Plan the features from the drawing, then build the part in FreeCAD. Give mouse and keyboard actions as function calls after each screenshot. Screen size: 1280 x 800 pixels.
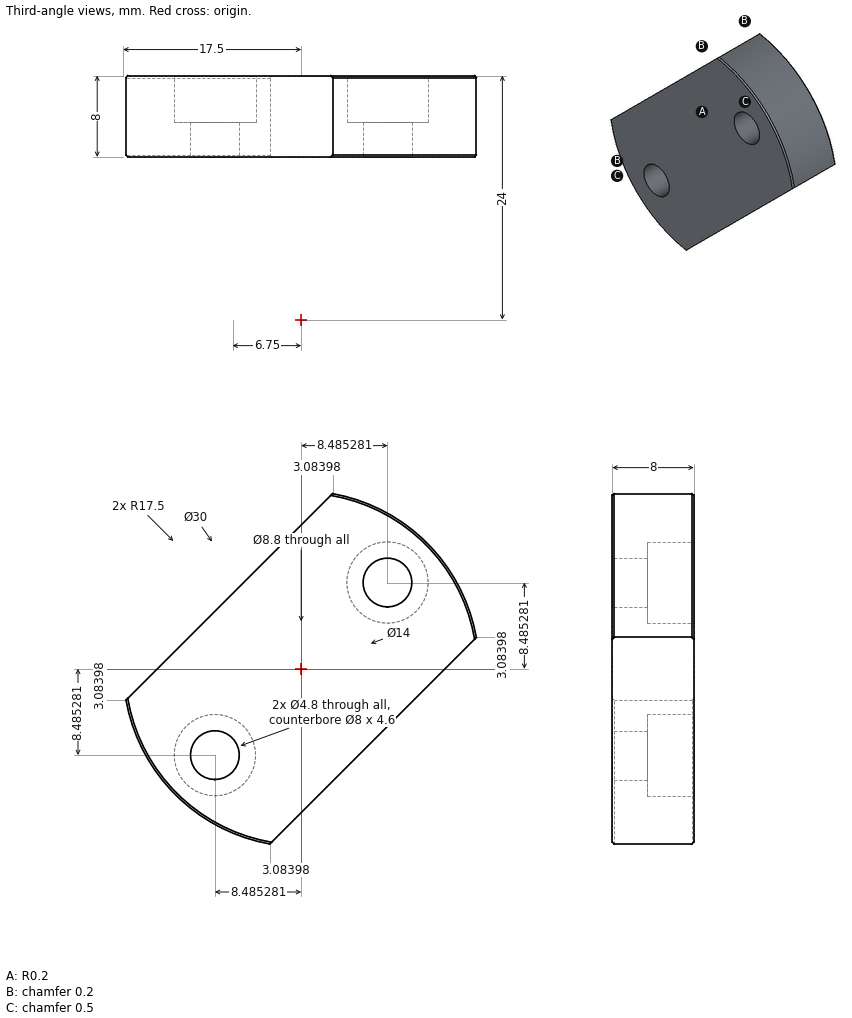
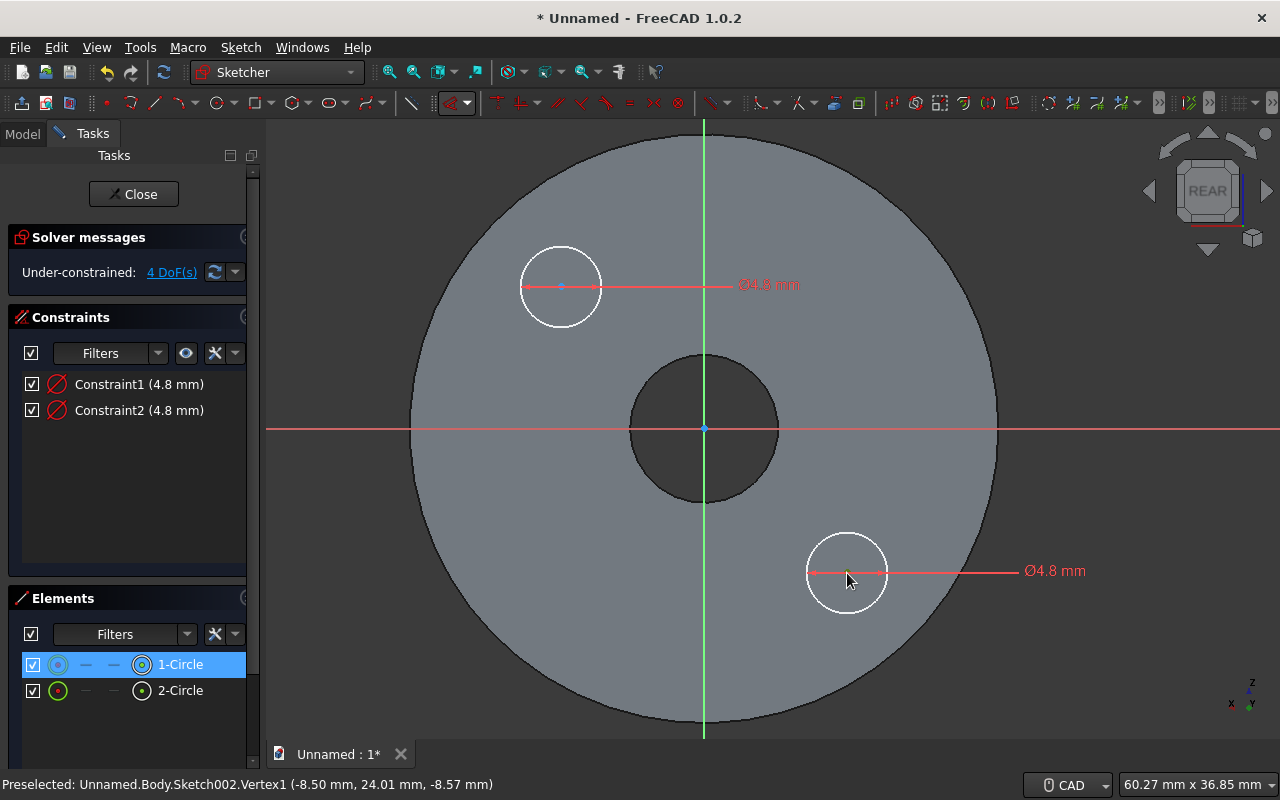
click(470, 104)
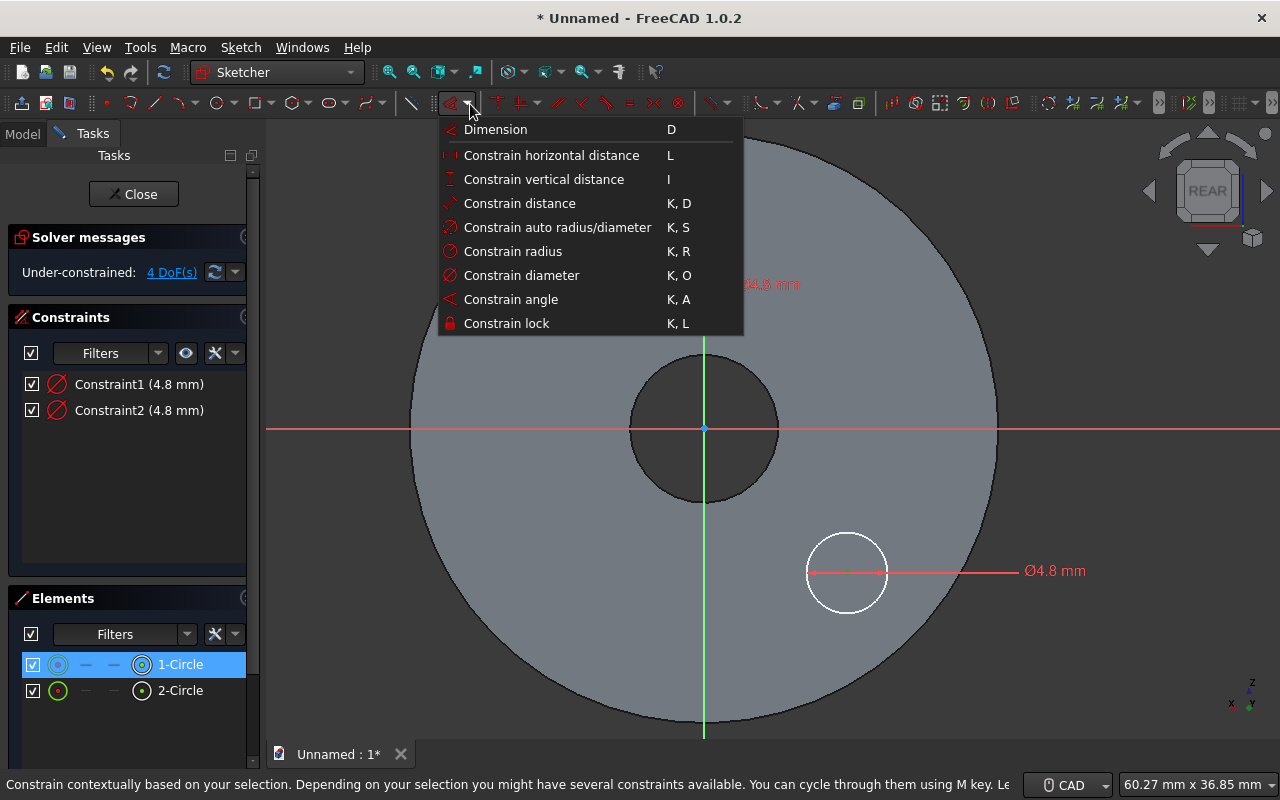
click(591, 155)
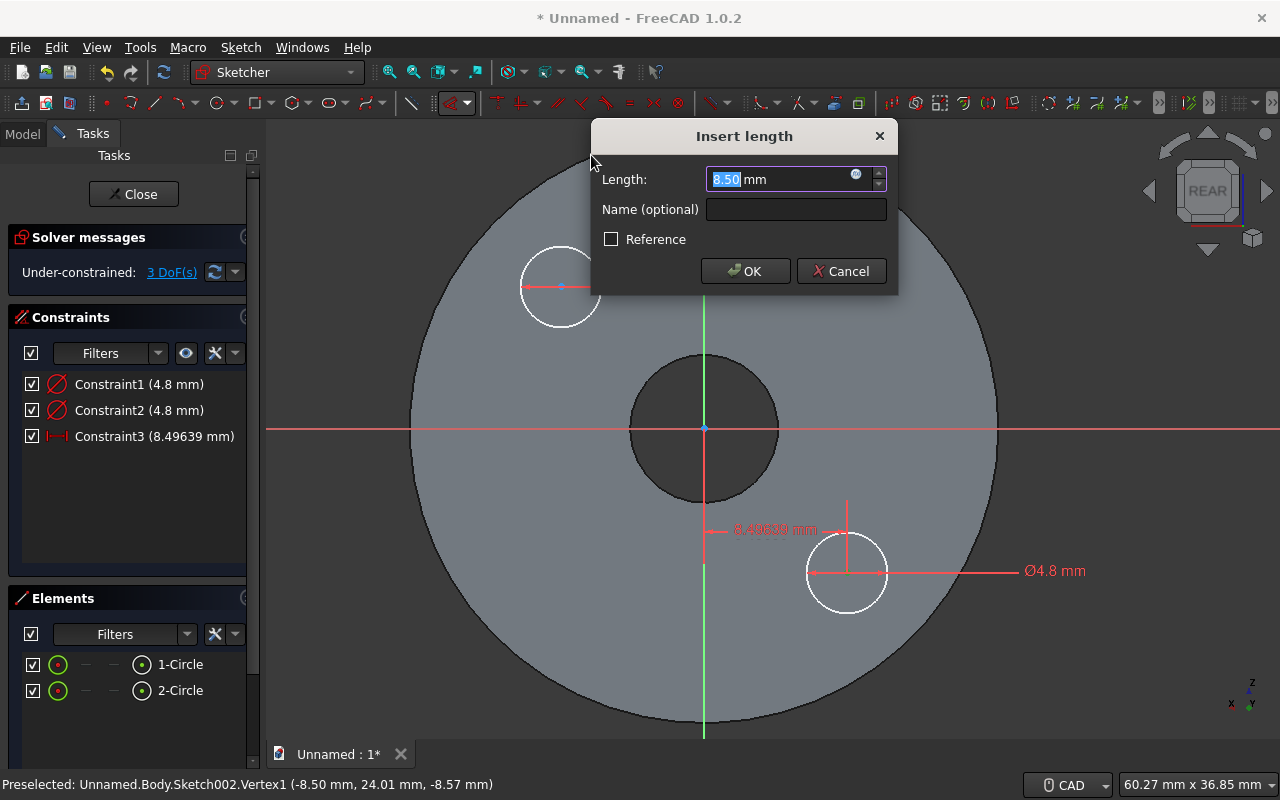
text(8.485281)
key(Return)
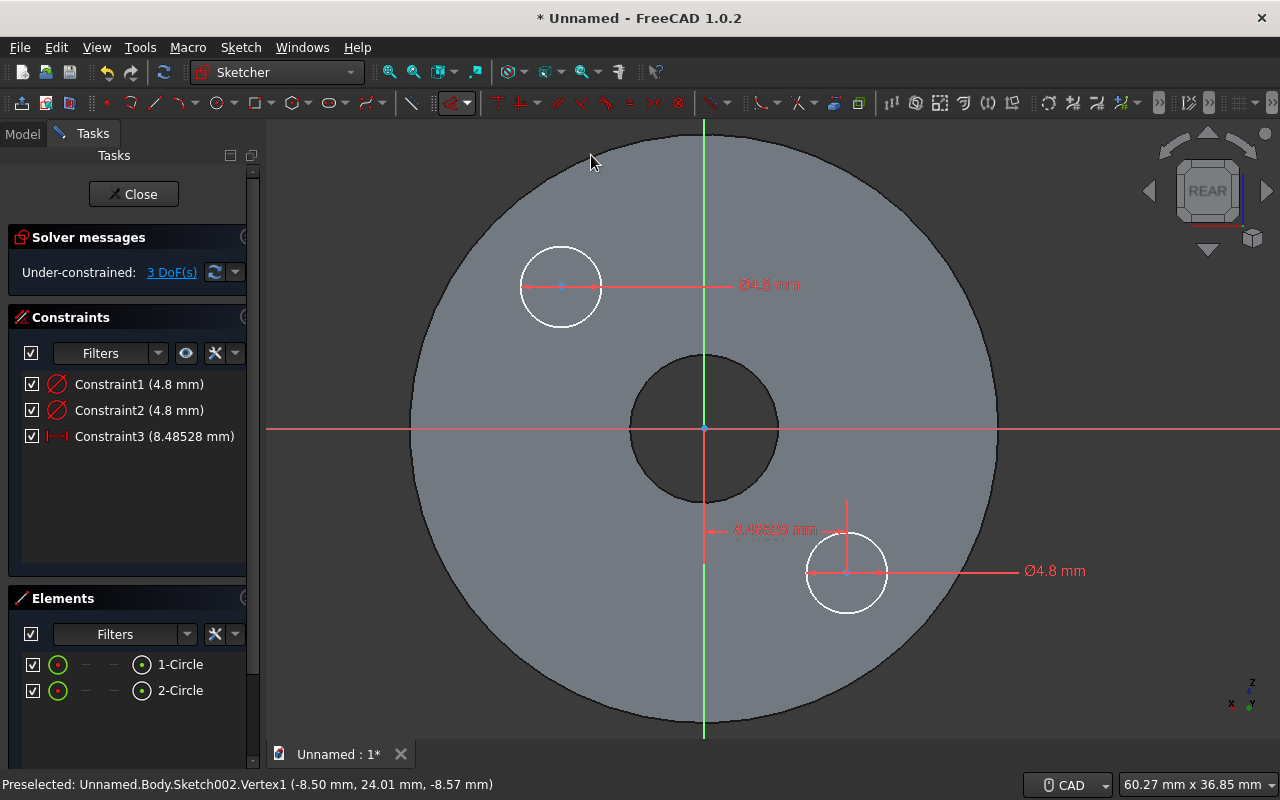
click(847, 573)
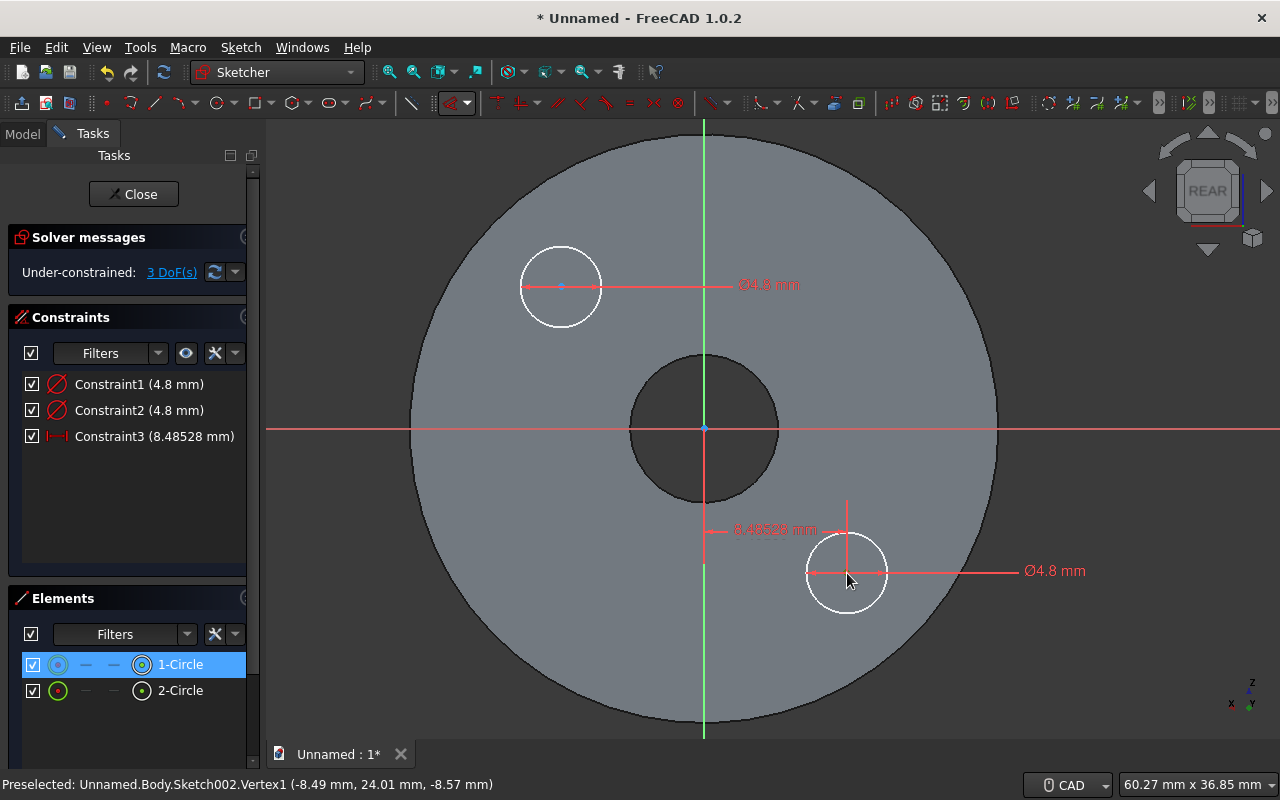
click(470, 104)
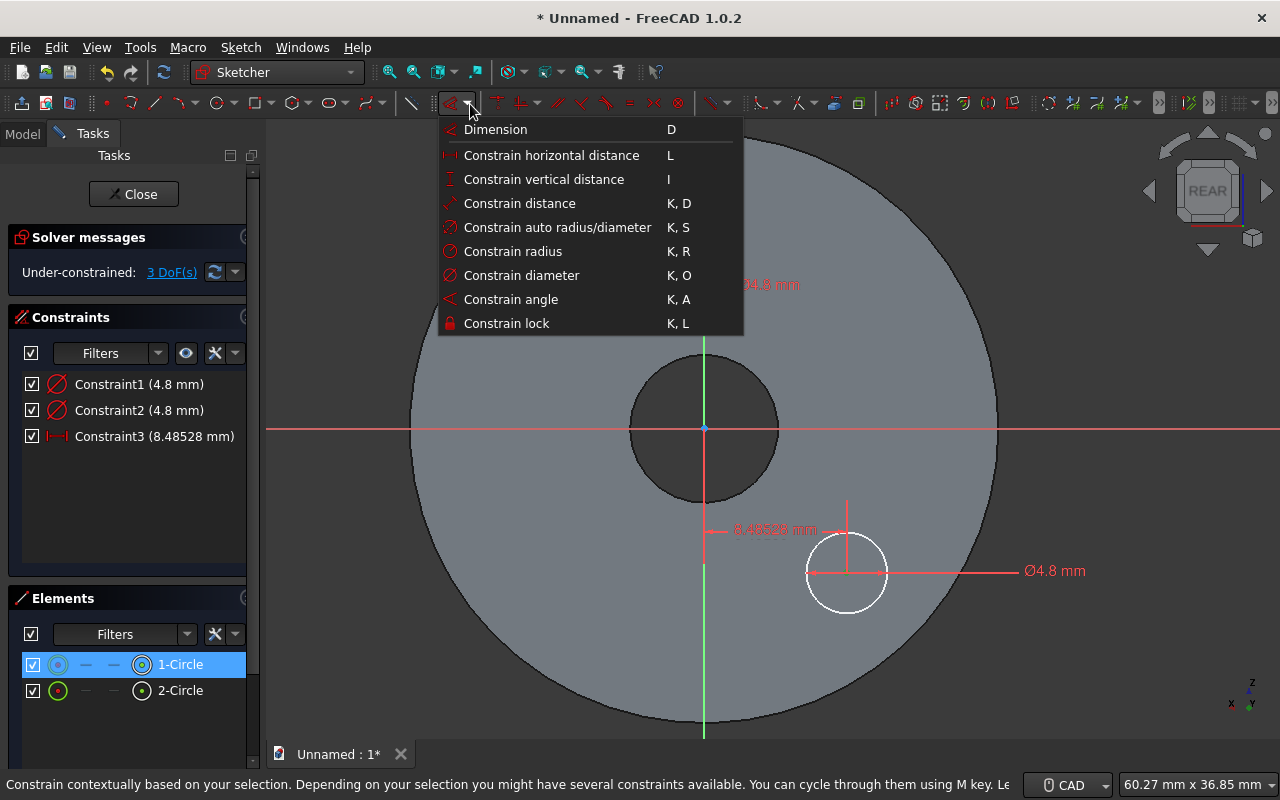
click(591, 179)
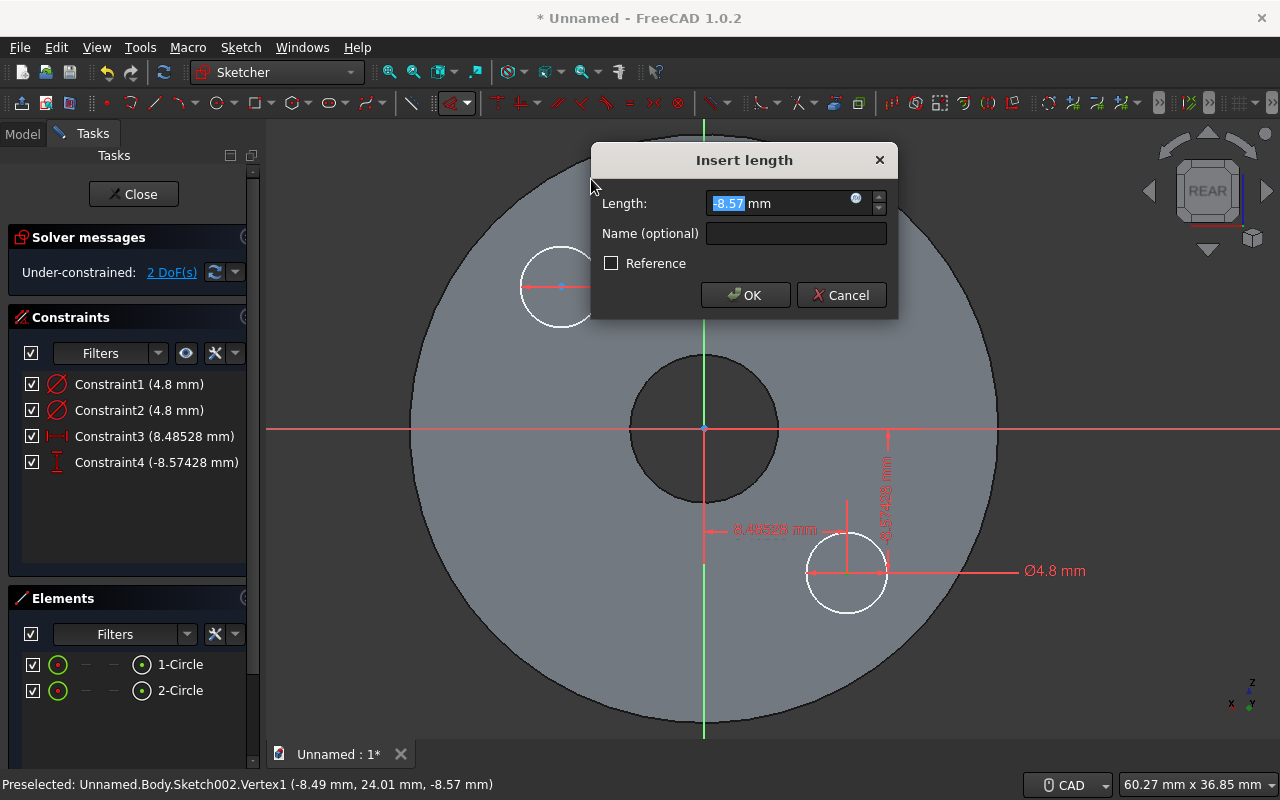
text(-8.485281)
key(Return)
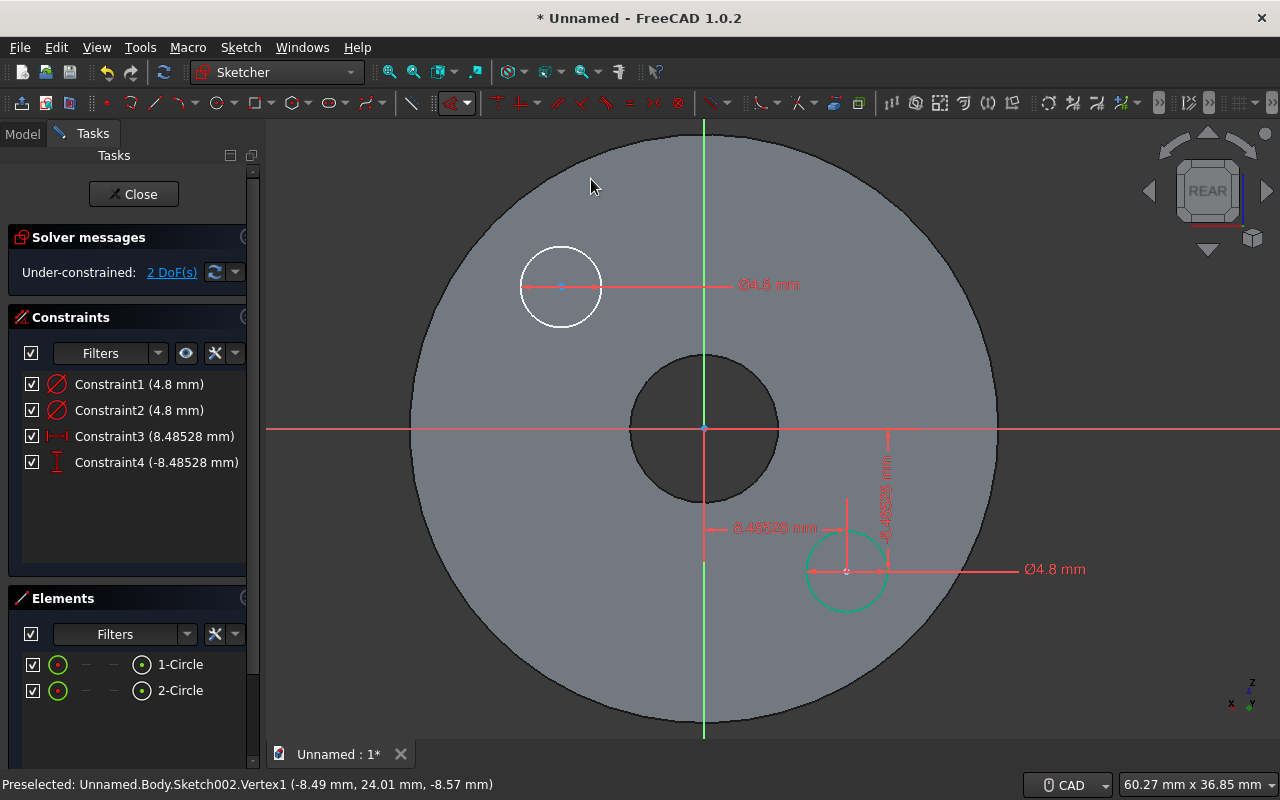
click(561, 287)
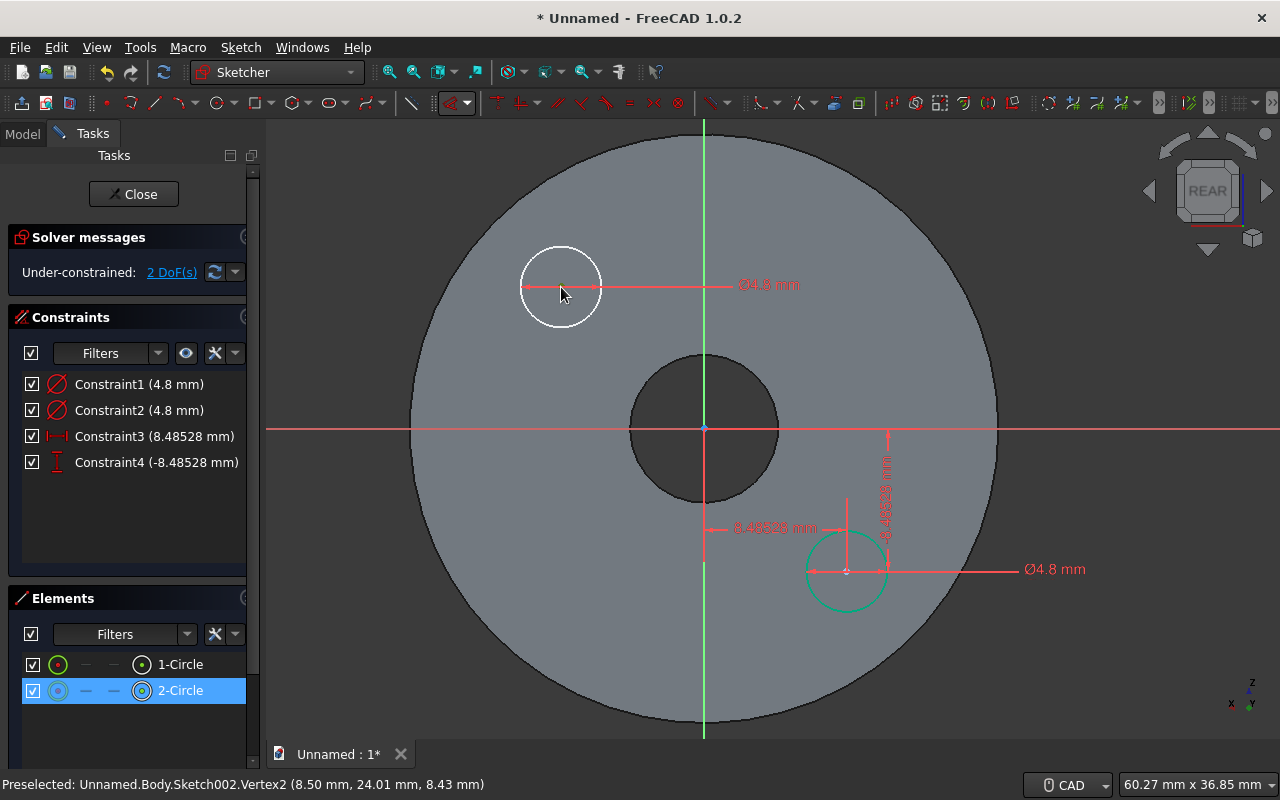
click(470, 104)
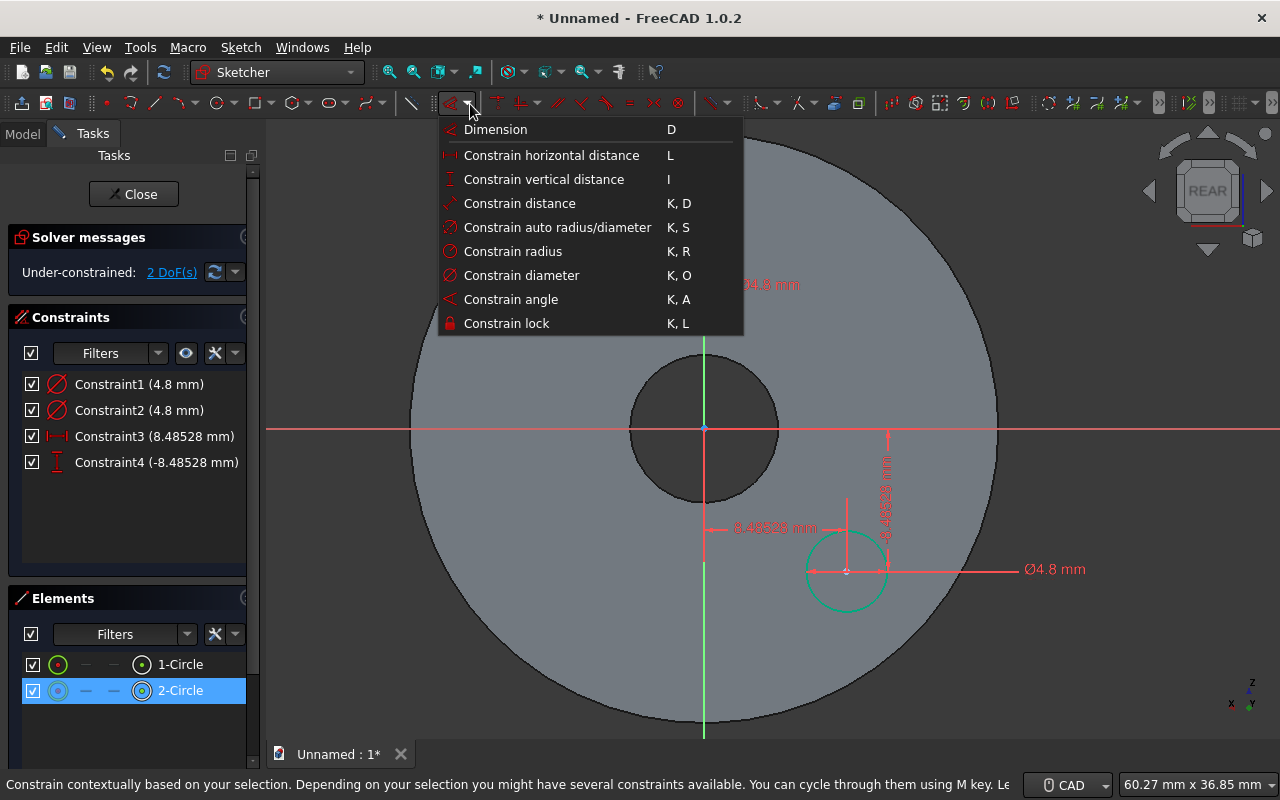
click(591, 155)